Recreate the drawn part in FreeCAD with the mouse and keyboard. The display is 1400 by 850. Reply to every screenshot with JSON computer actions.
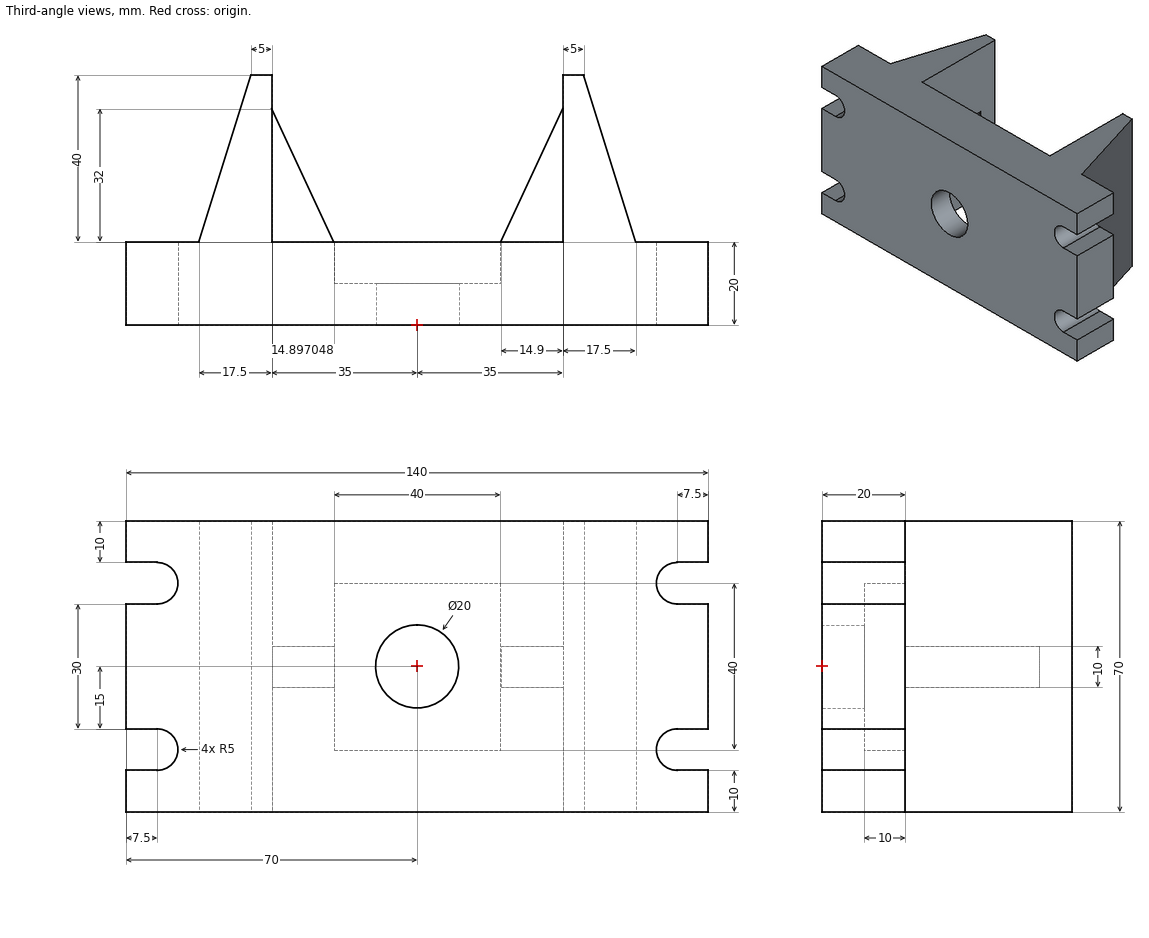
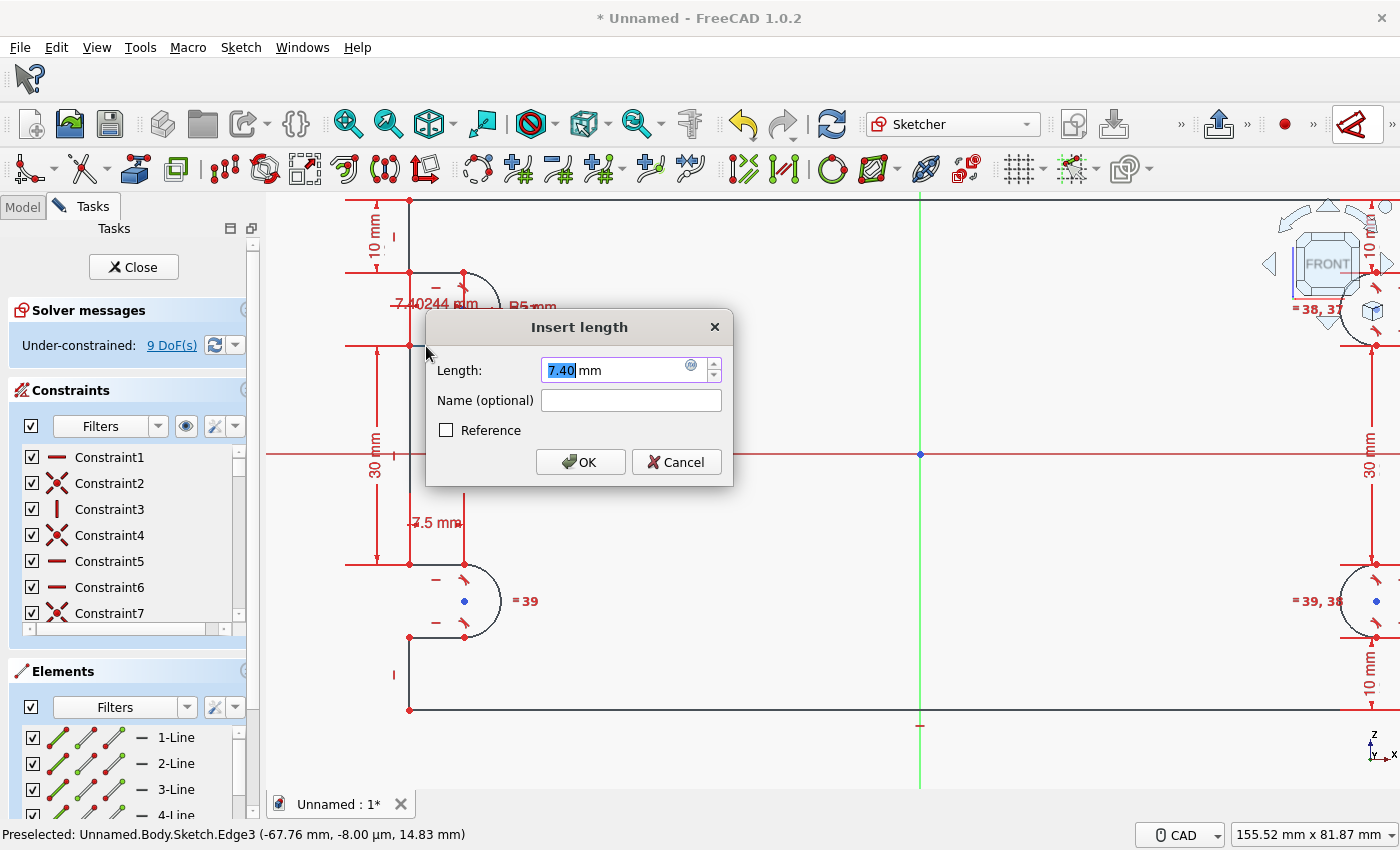
{"action": "type", "text": "7.5"}
{"action": "key", "text": "Return"}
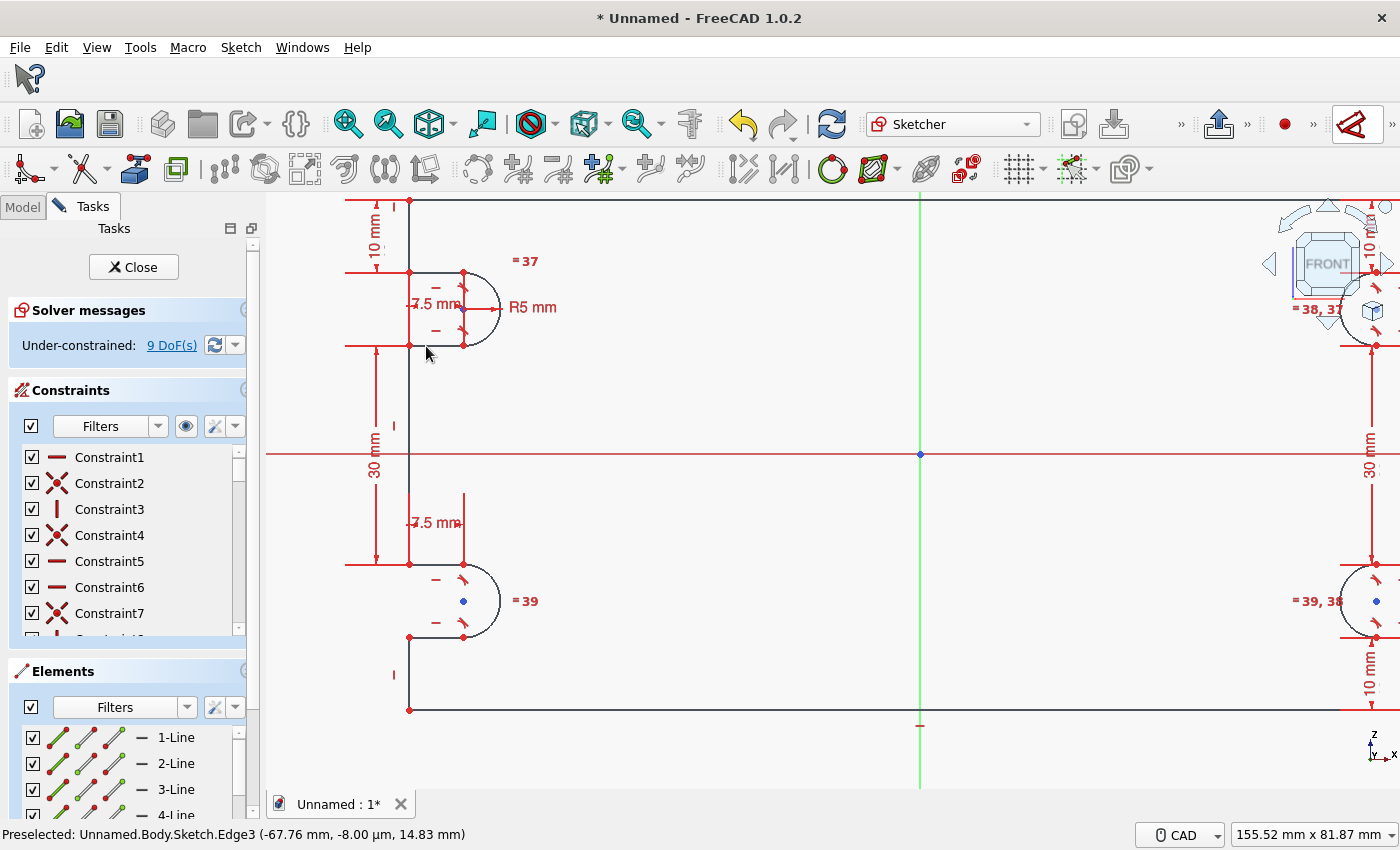
{"action": "left_click", "coordinate": [447, 273]}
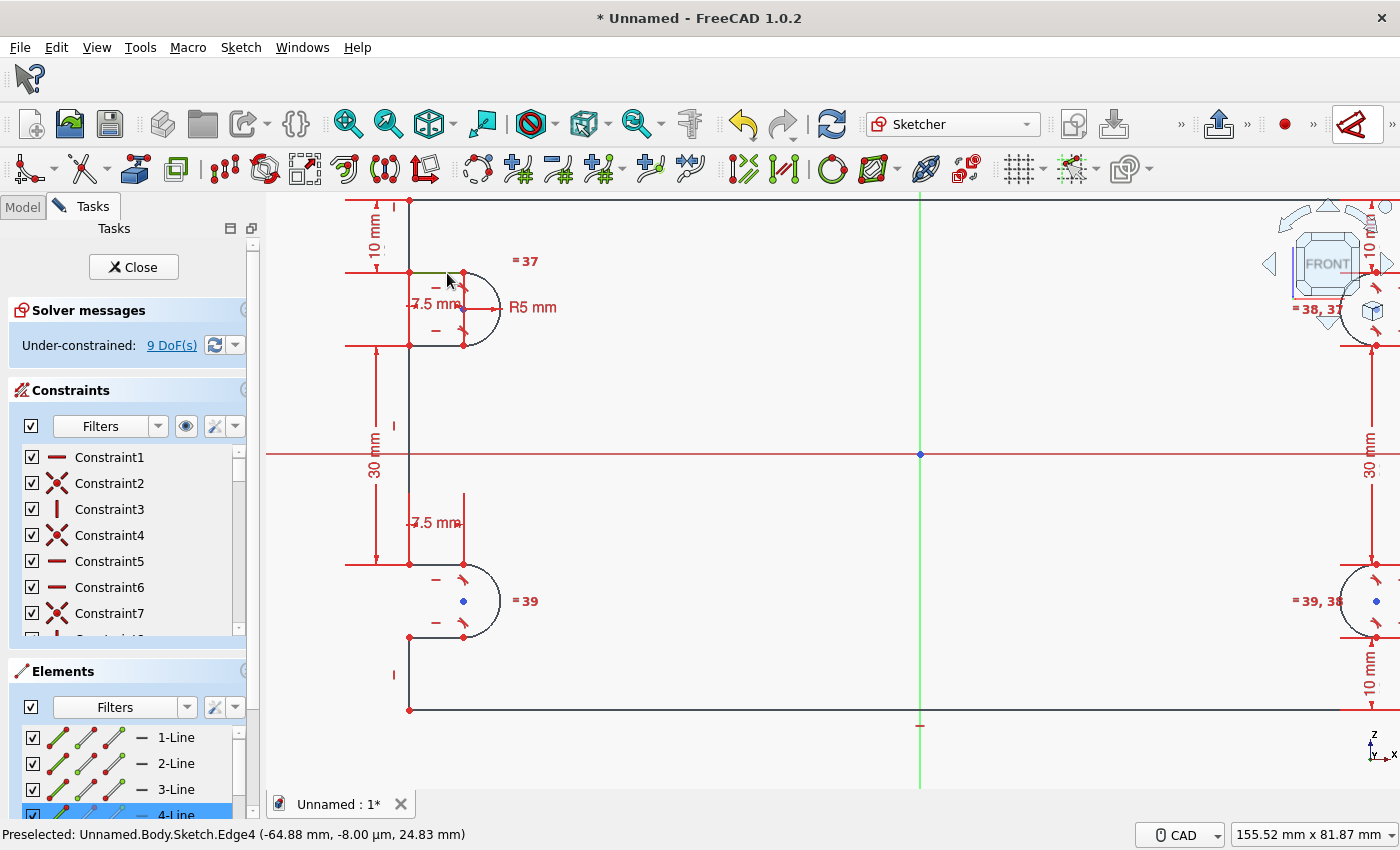
{"action": "left_click", "coordinate": [1378, 124]}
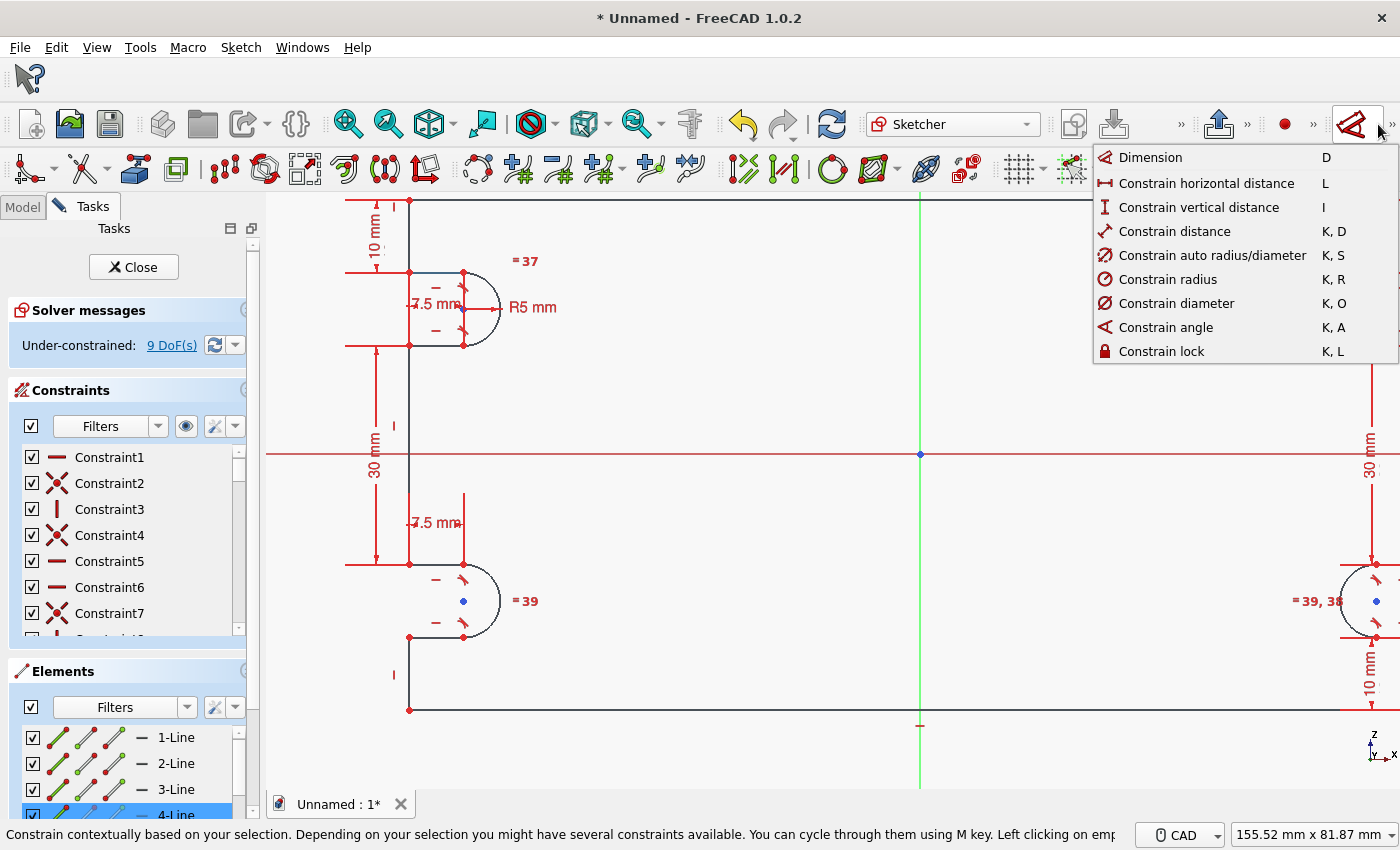
{"action": "left_click", "coordinate": [1246, 183]}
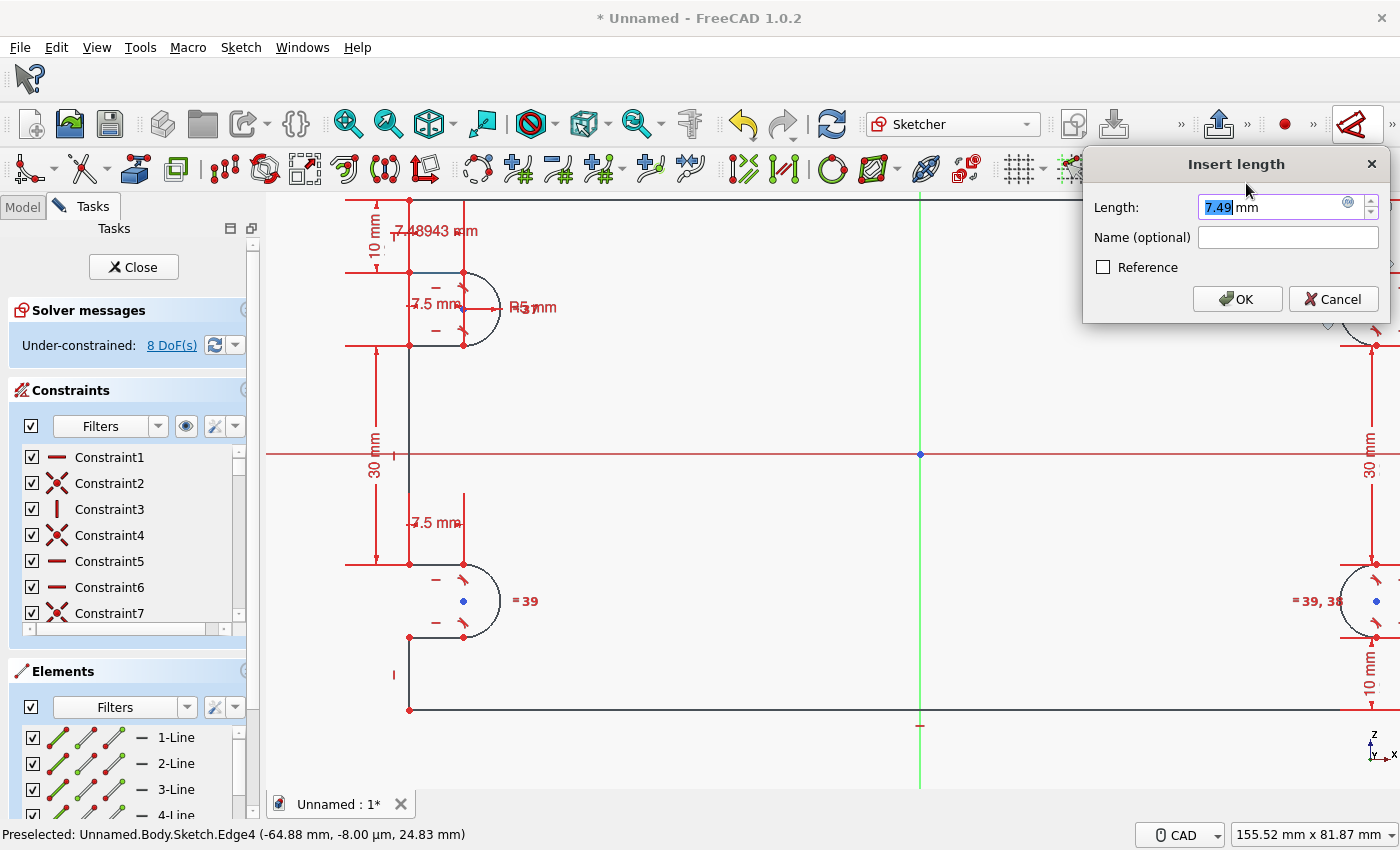
{"action": "type", "text": "7.5"}
{"action": "key", "text": "Return"}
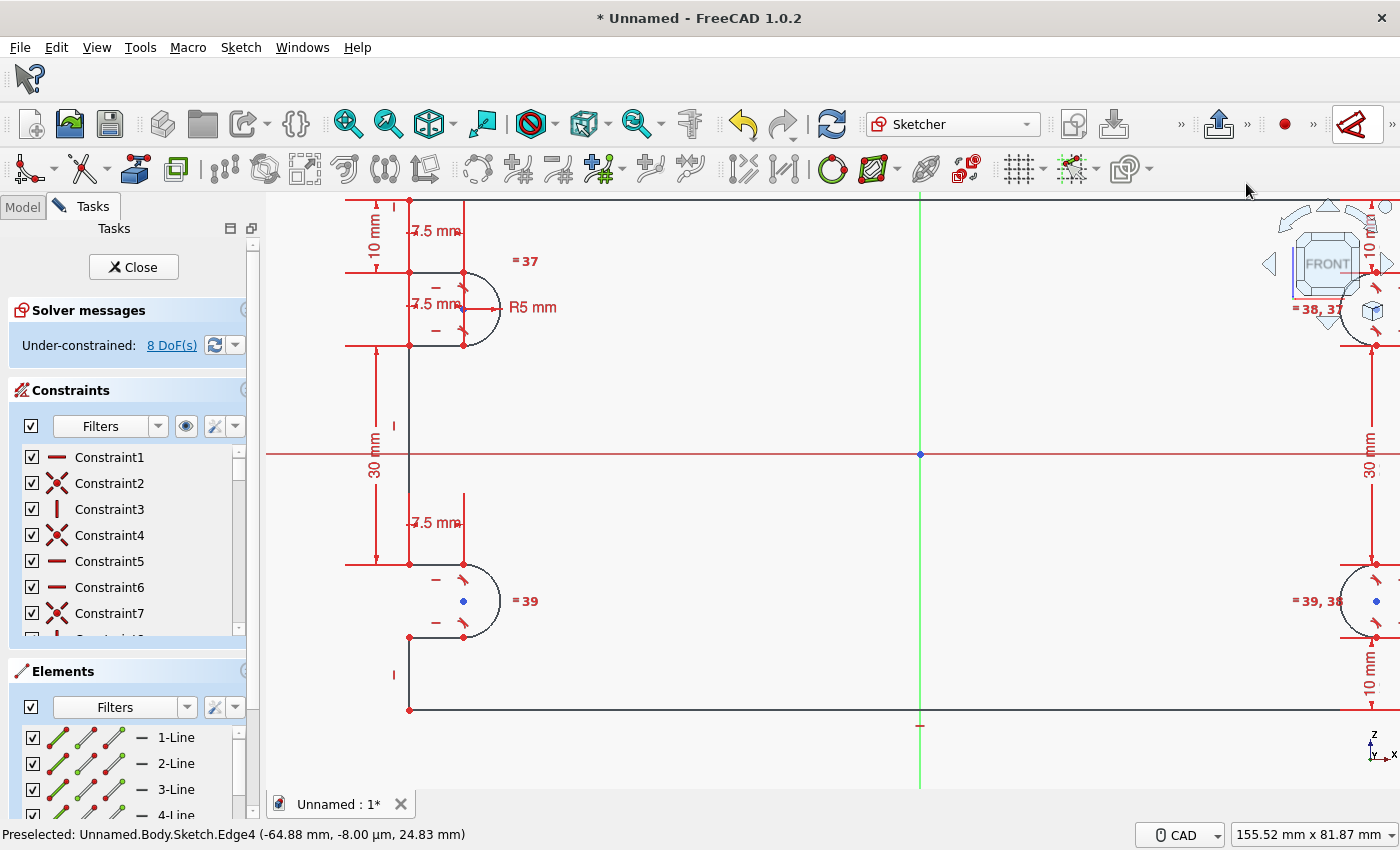
{"action": "scroll", "coordinate": [448, 565], "scroll_direction": "down", "scroll_amount": 2}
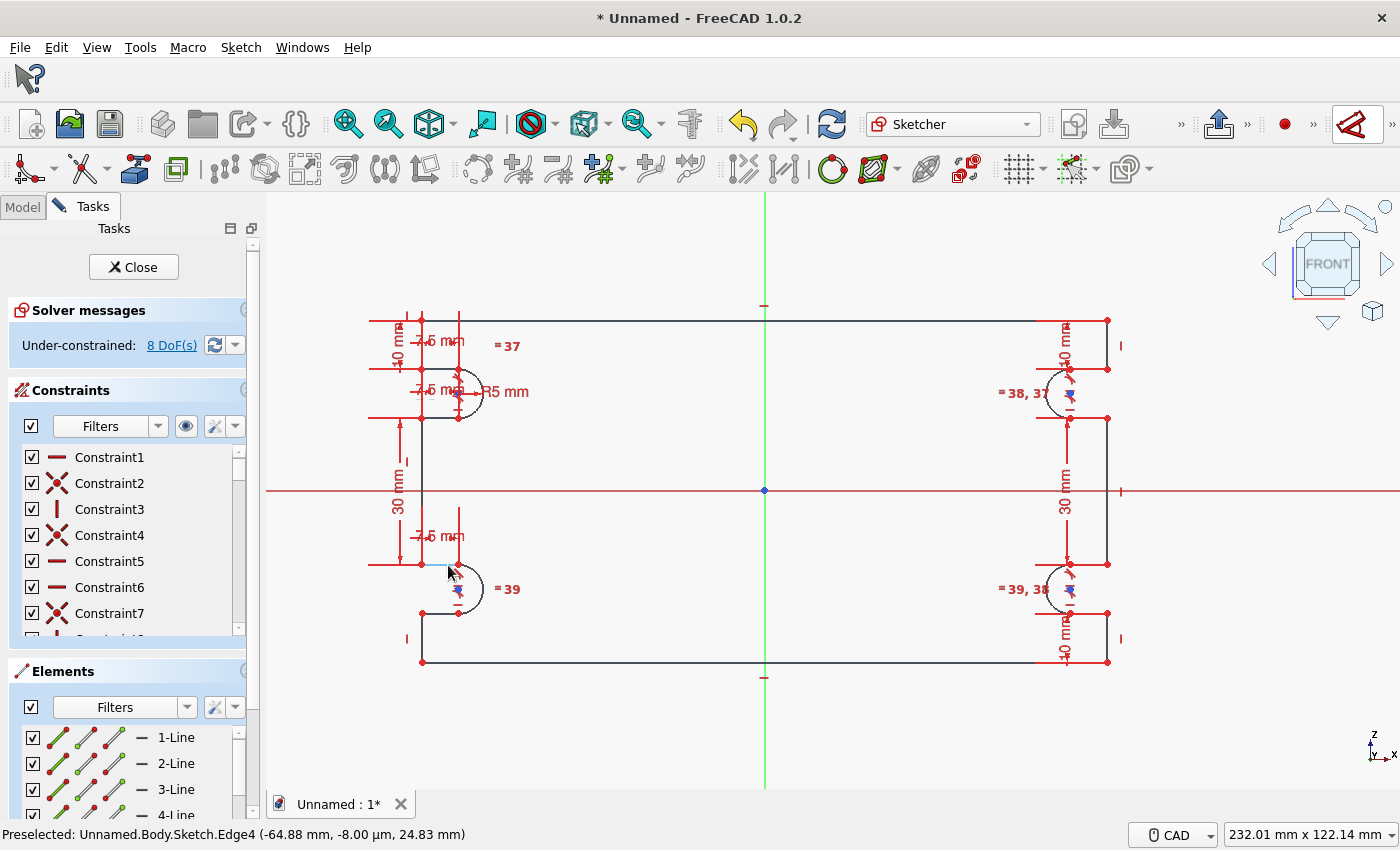
{"action": "left_click", "coordinate": [627, 321]}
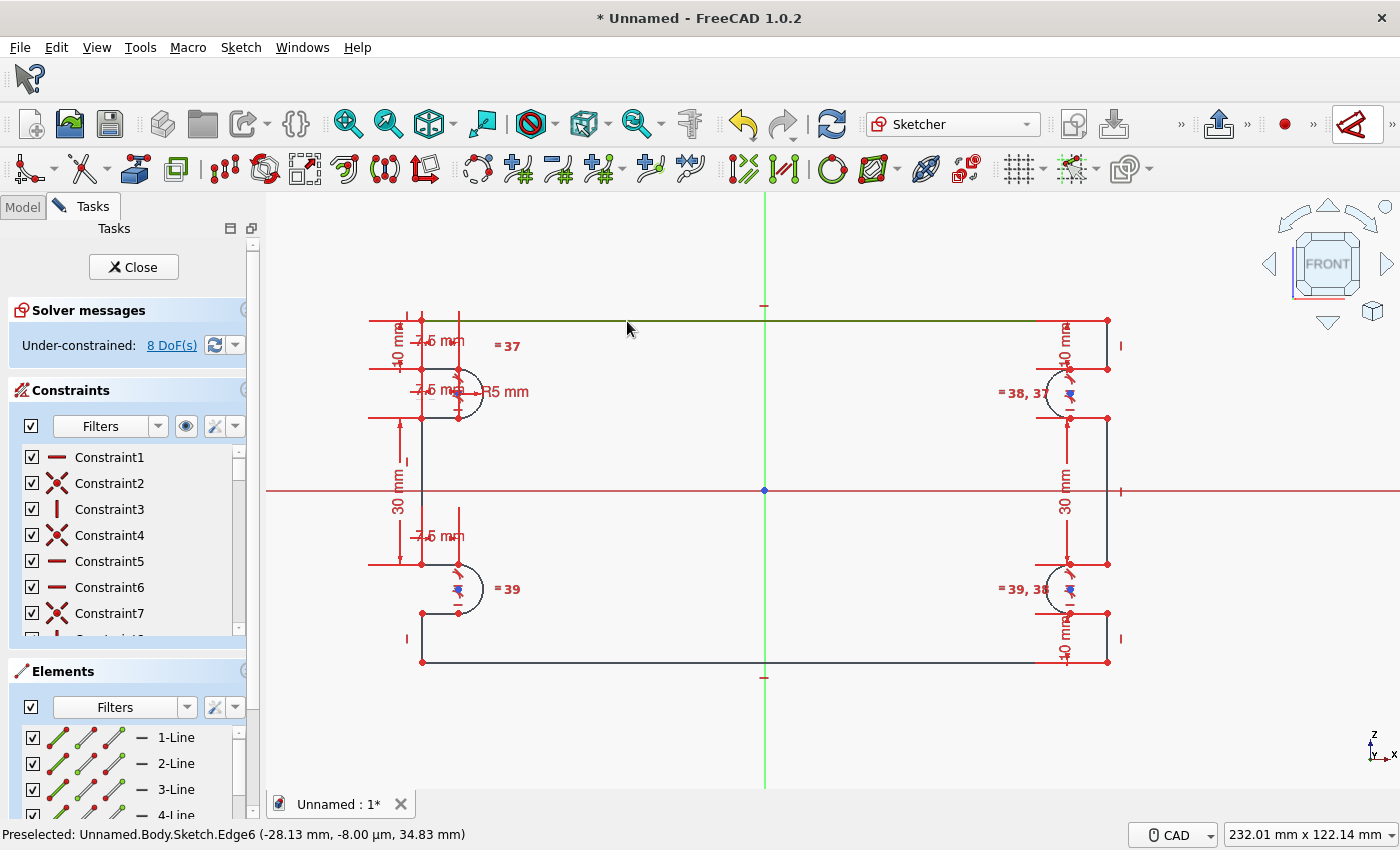
{"action": "key", "text": "l"}